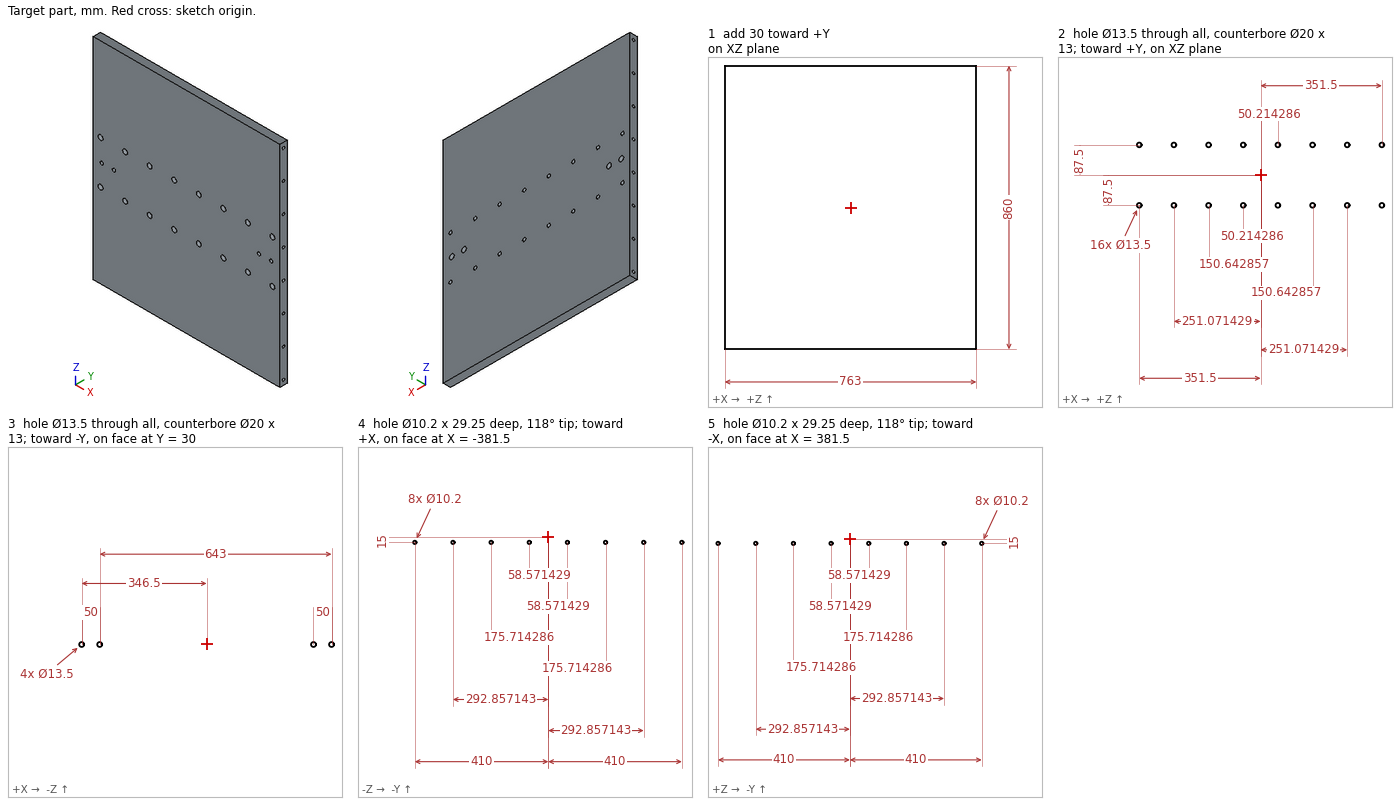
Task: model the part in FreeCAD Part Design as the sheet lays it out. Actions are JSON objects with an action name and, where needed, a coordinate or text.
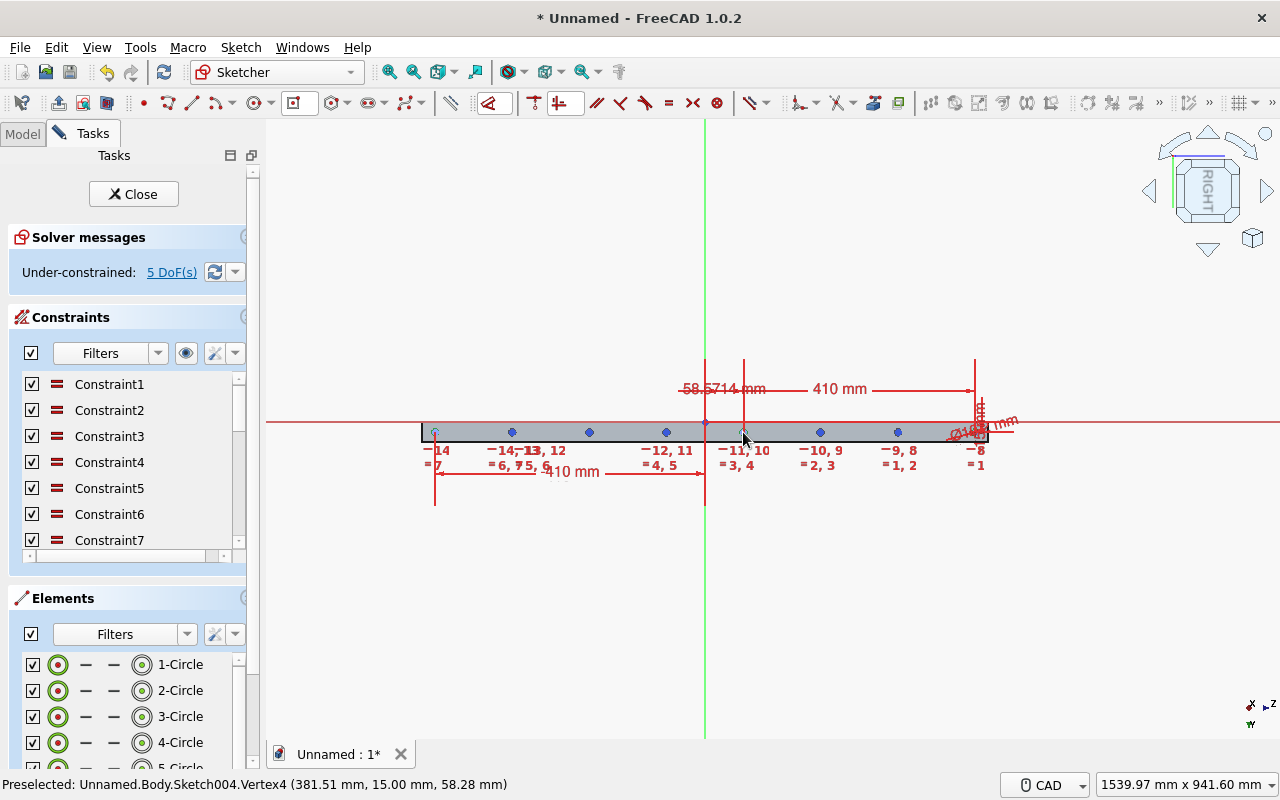
{"action": "left_click", "coordinate": [666, 432]}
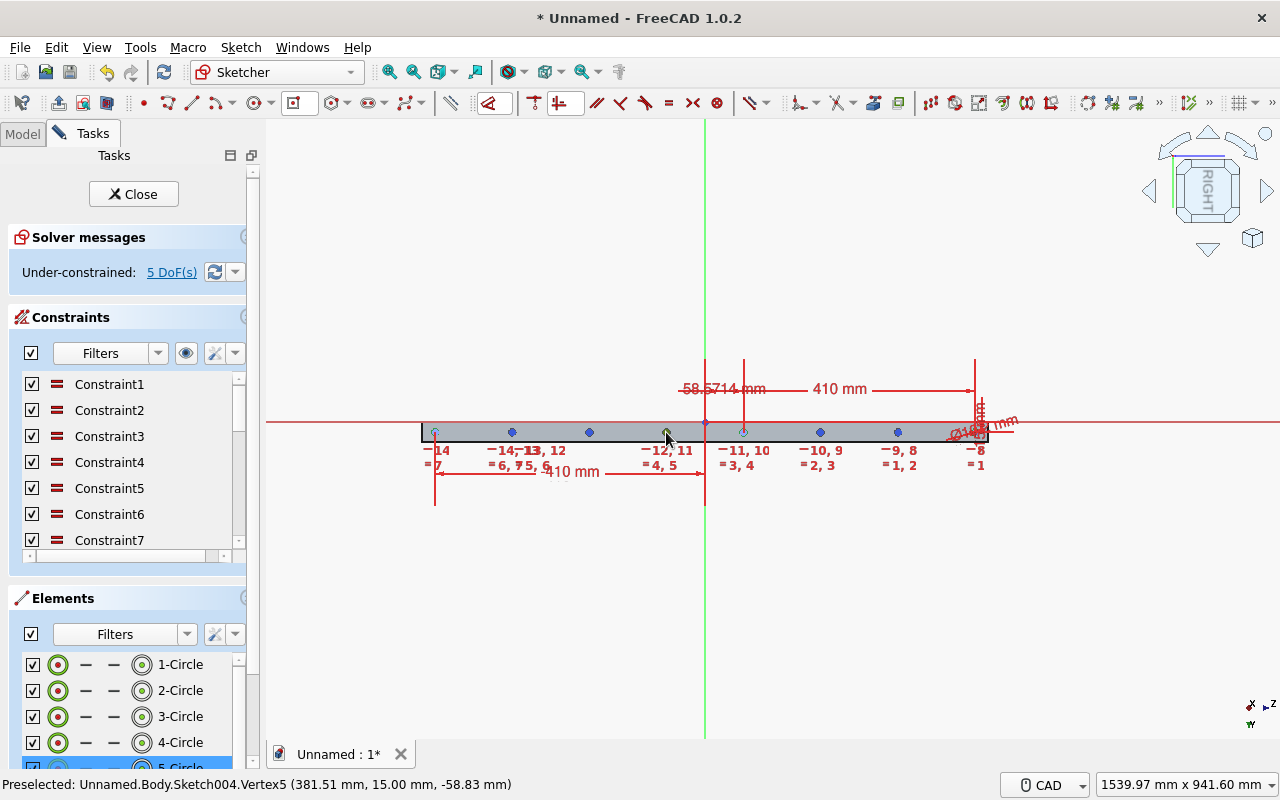
{"action": "left_click", "coordinate": [506, 104]}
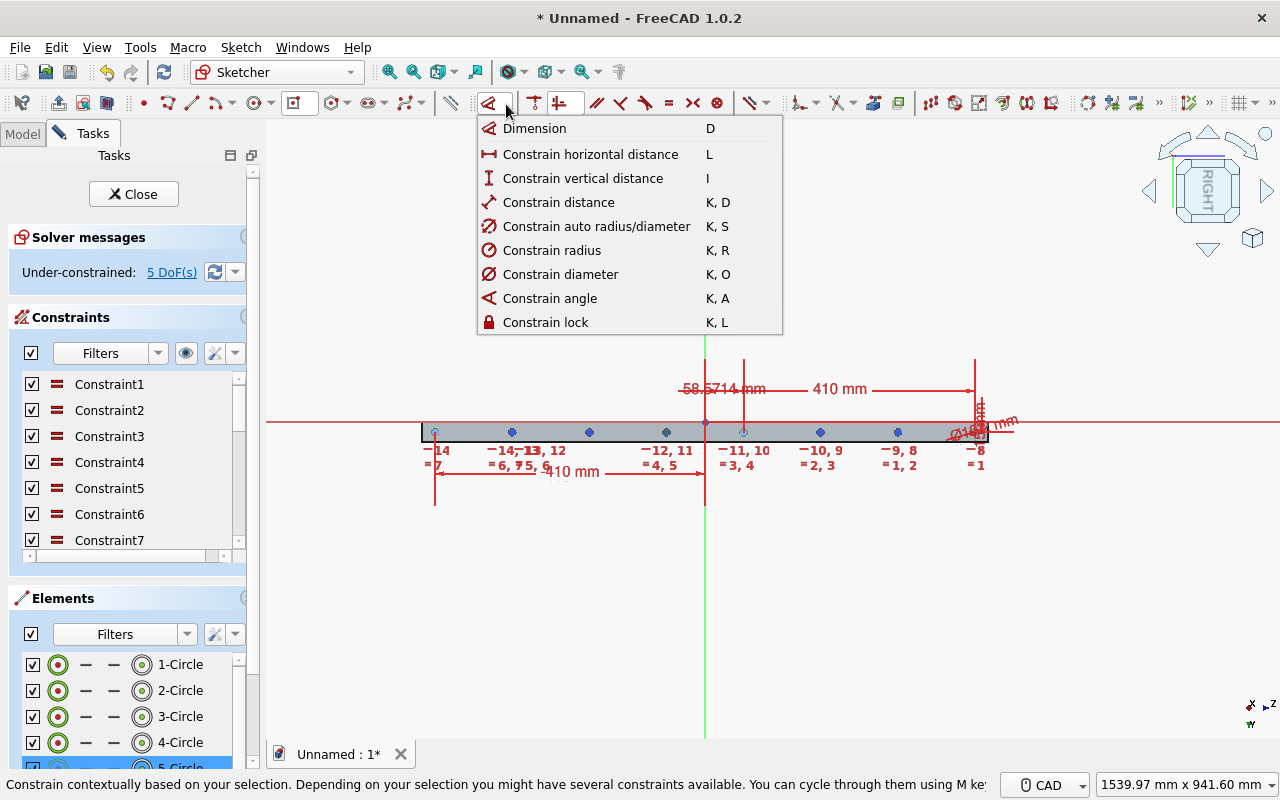
{"action": "left_click", "coordinate": [630, 154]}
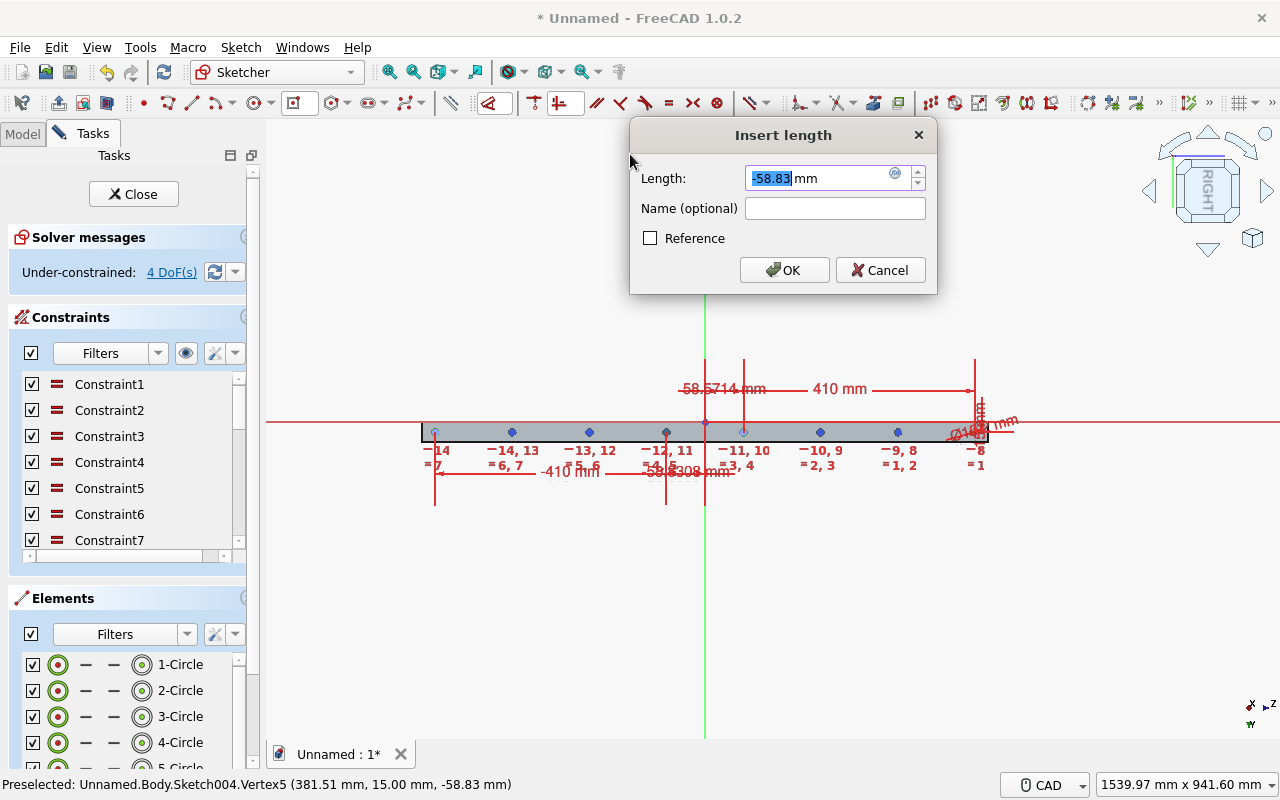
{"action": "type", "text": "-58.571429"}
{"action": "key", "text": "Return"}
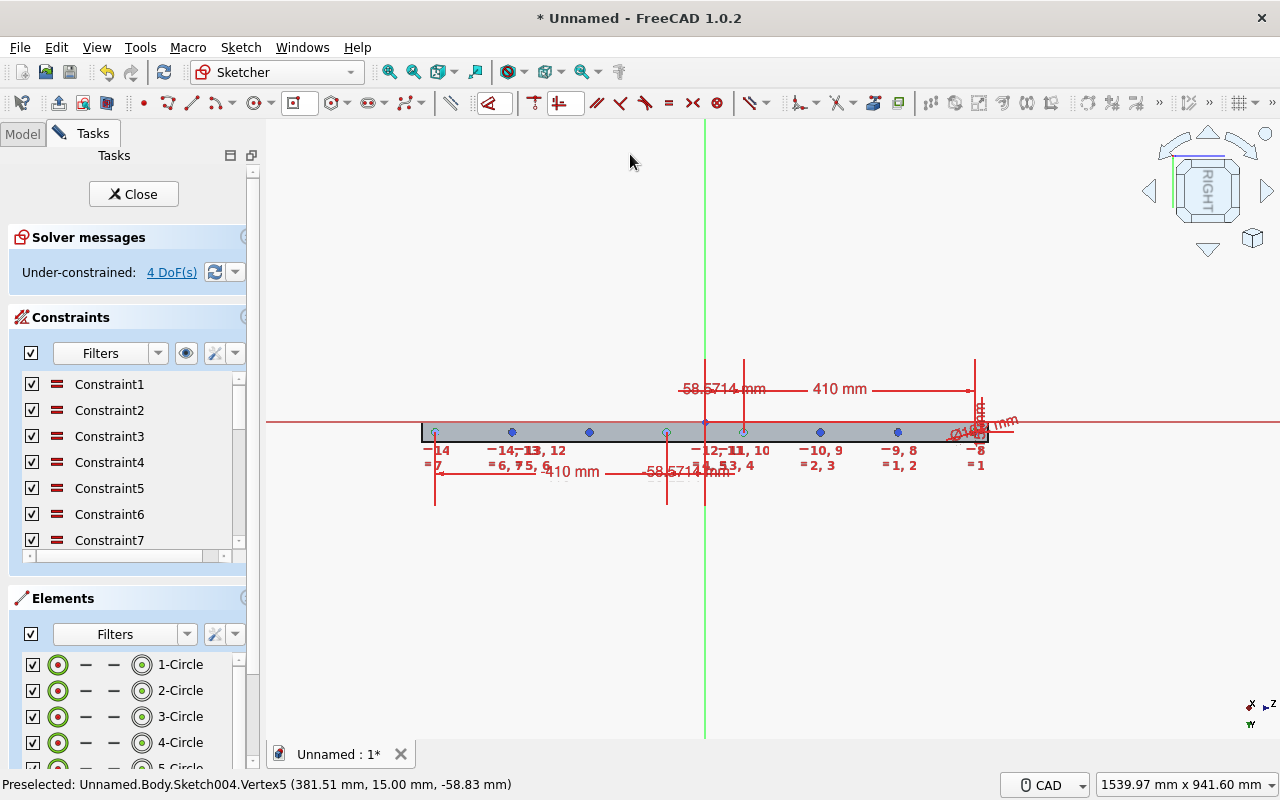
{"action": "left_click", "coordinate": [898, 432]}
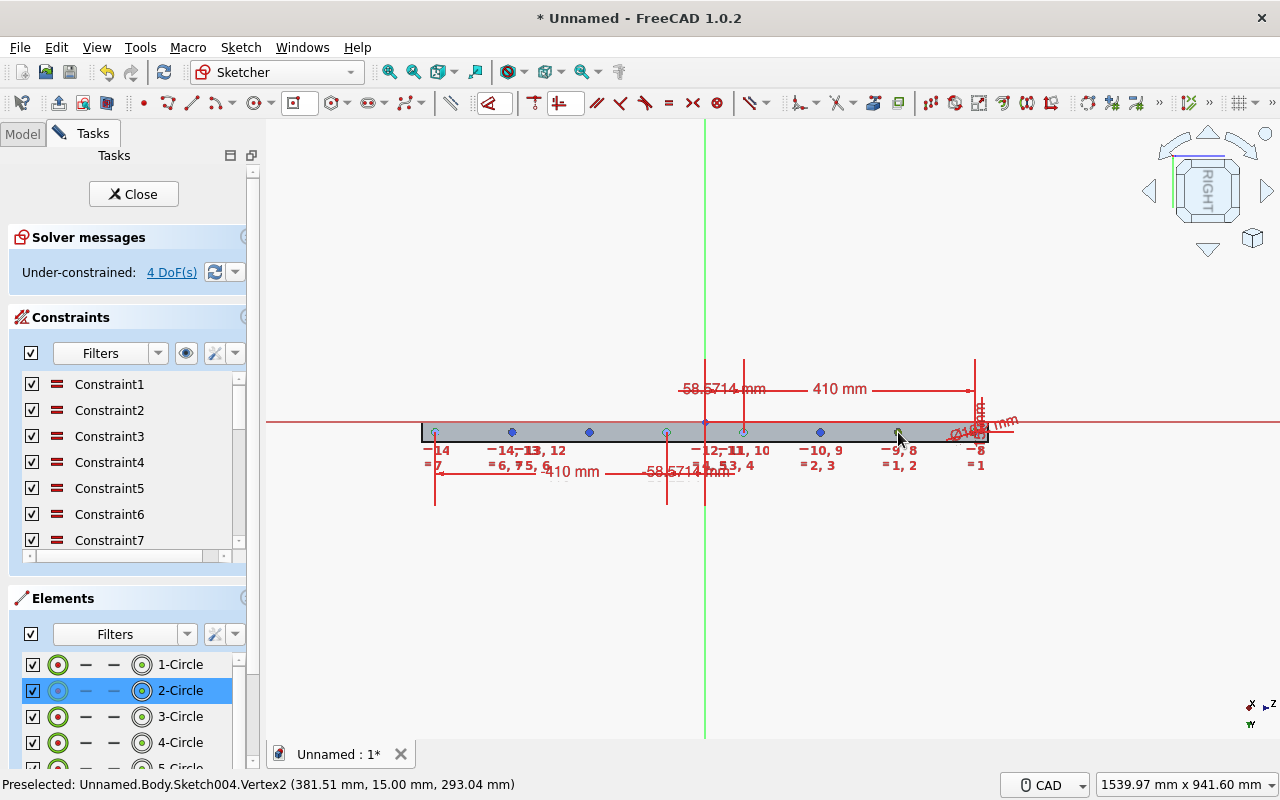
{"action": "left_click", "coordinate": [506, 104]}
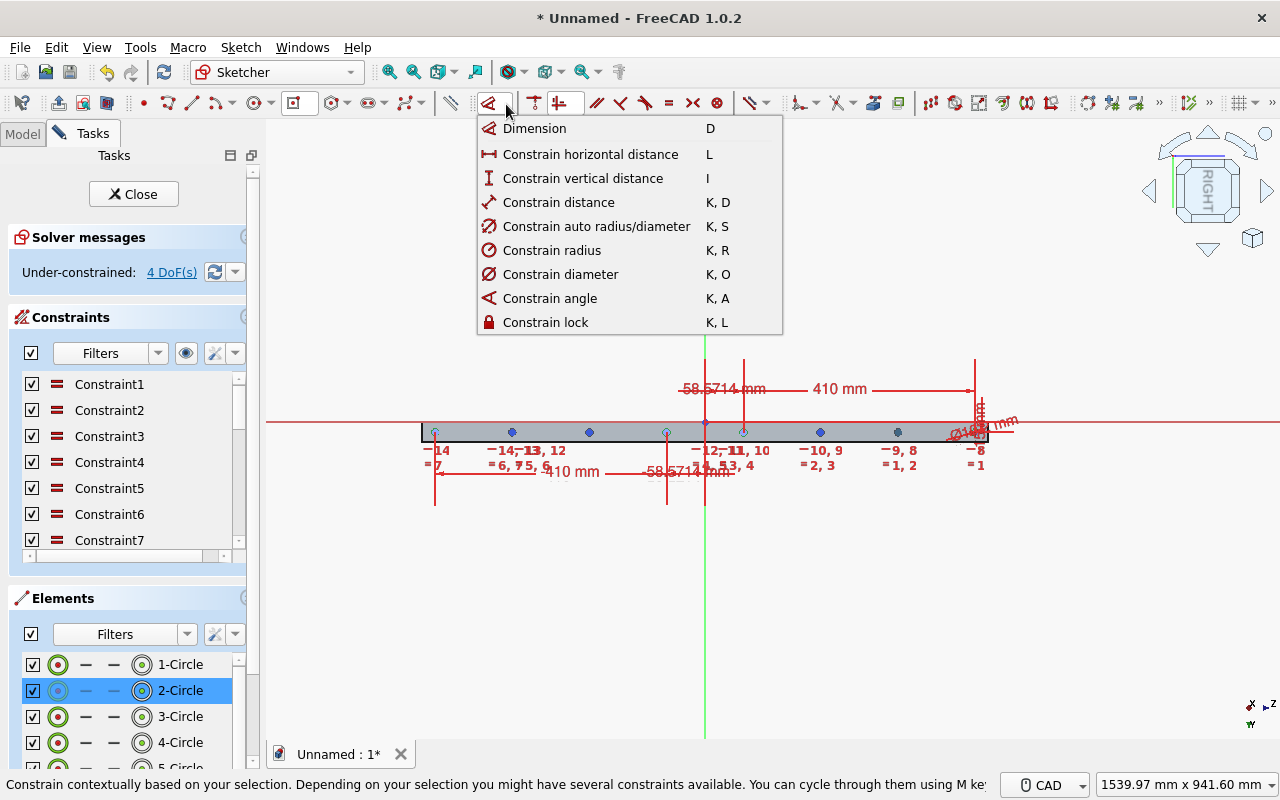
{"action": "left_click", "coordinate": [630, 154]}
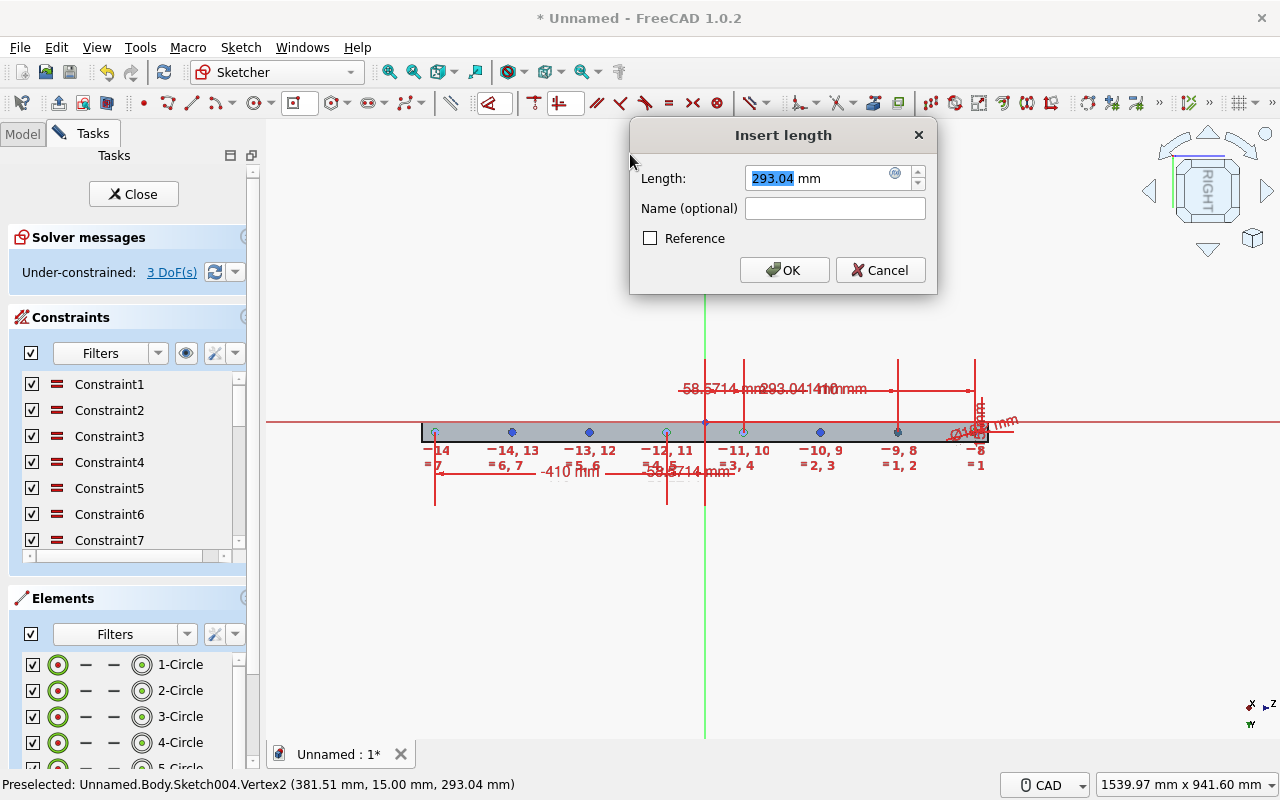
{"action": "type", "text": "292.857143"}
{"action": "key", "text": "Return"}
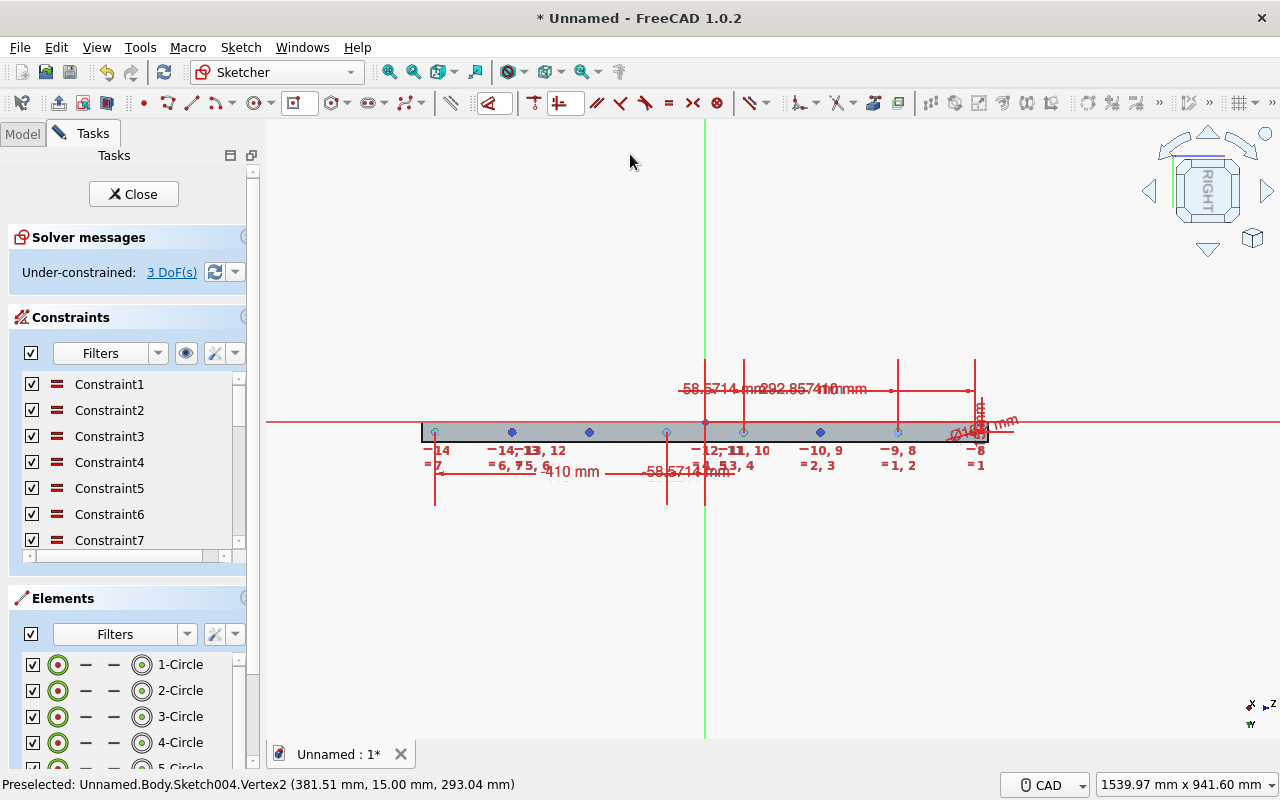
{"action": "left_click", "coordinate": [821, 432]}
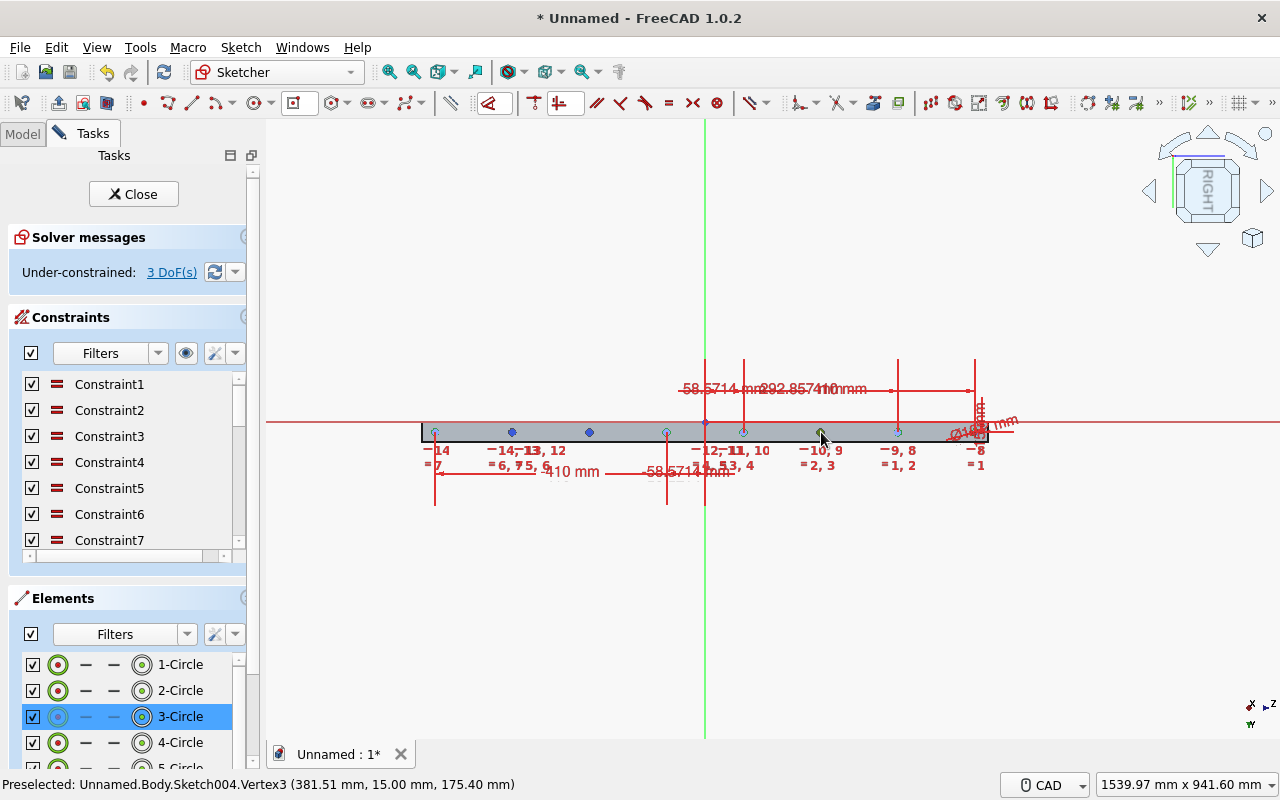
{"action": "left_click", "coordinate": [506, 104]}